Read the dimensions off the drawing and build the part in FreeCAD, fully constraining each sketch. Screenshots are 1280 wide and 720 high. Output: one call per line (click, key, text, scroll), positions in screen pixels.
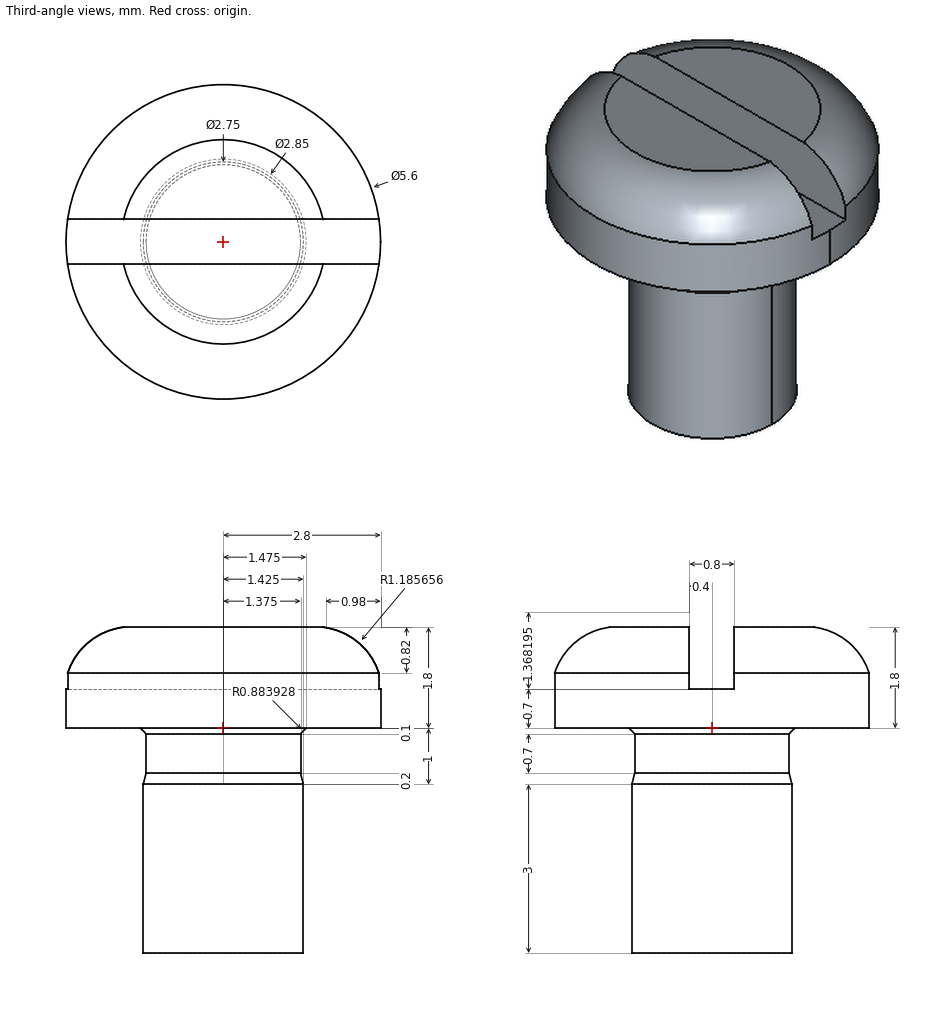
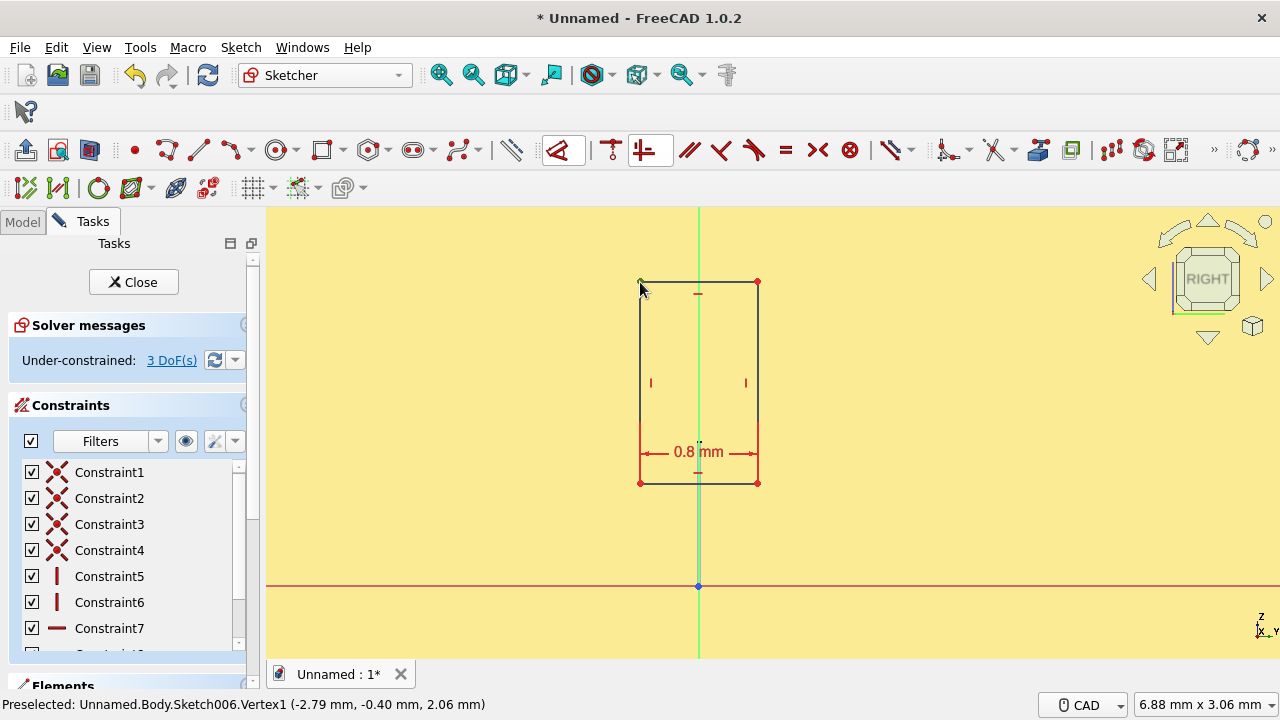
click(580, 150)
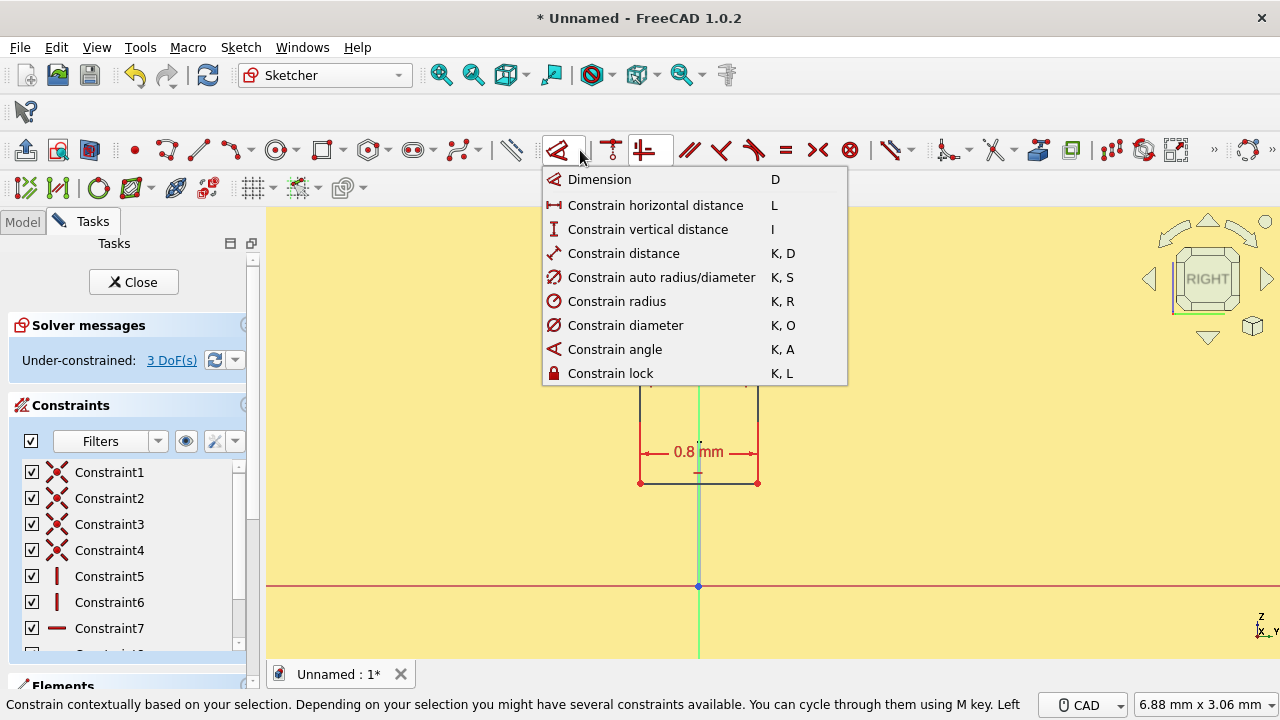
click(695, 205)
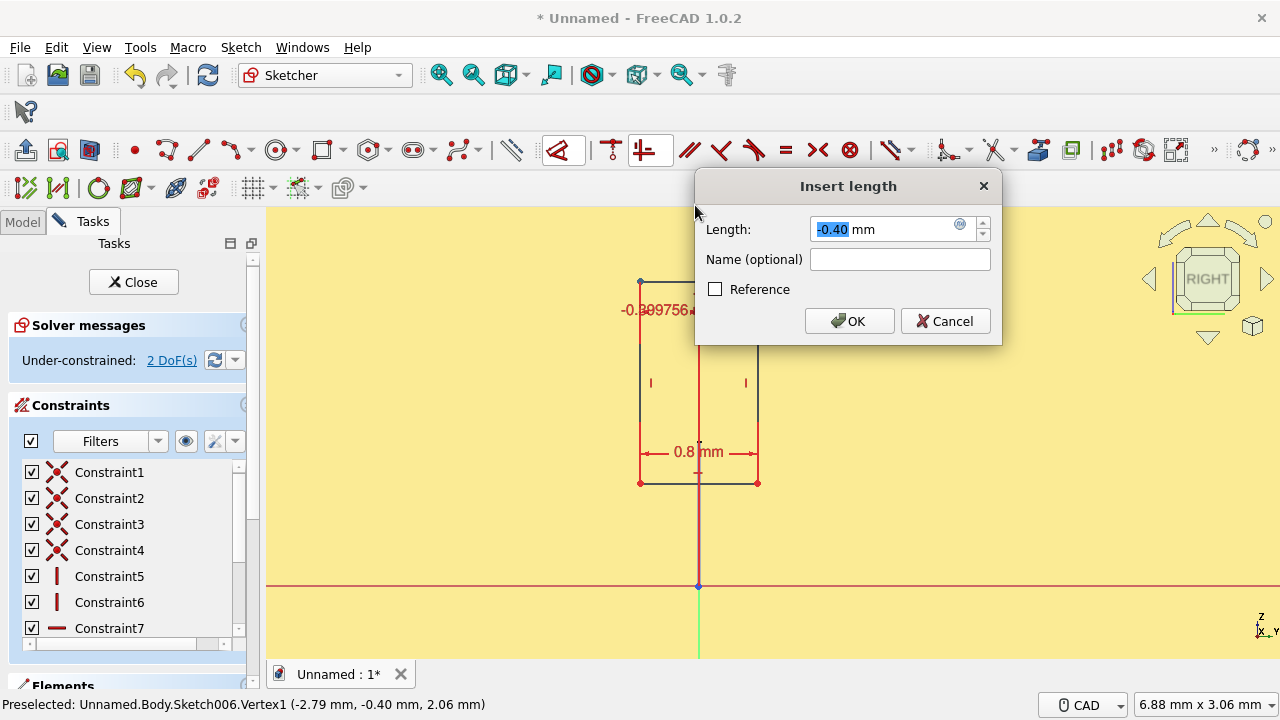
text(-0.4)
key(Return)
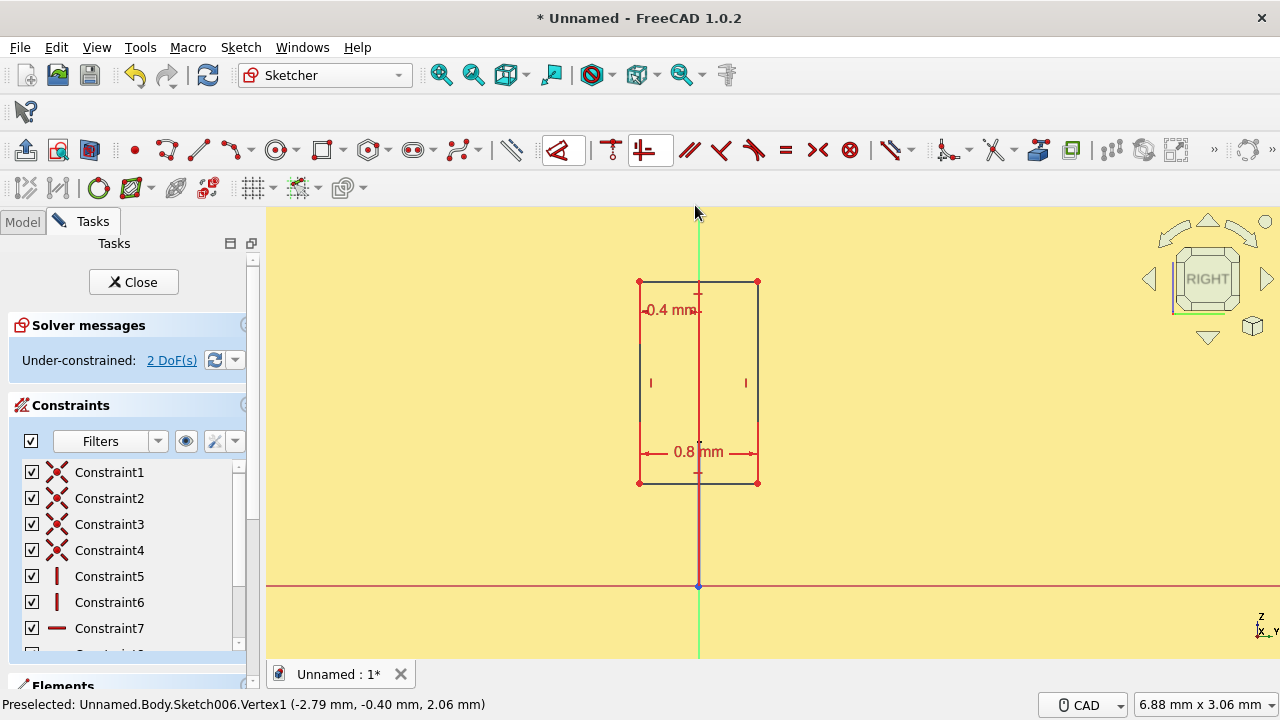
click(640, 484)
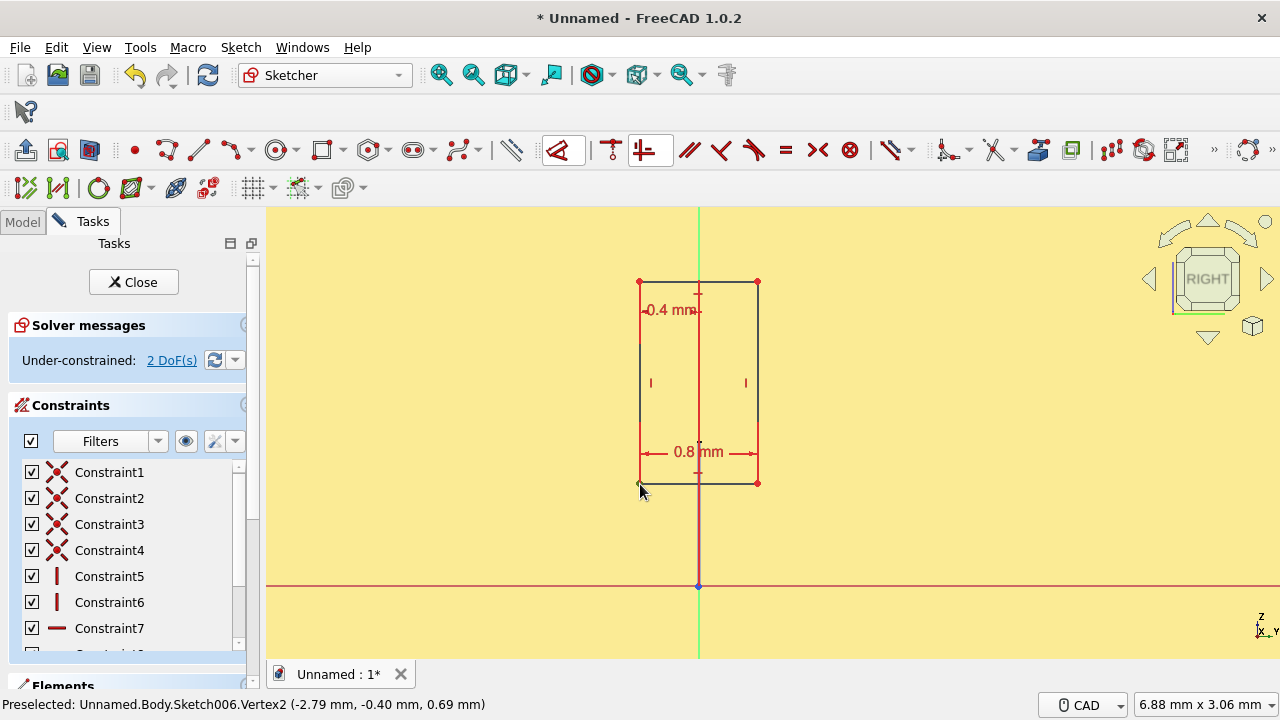
click(580, 150)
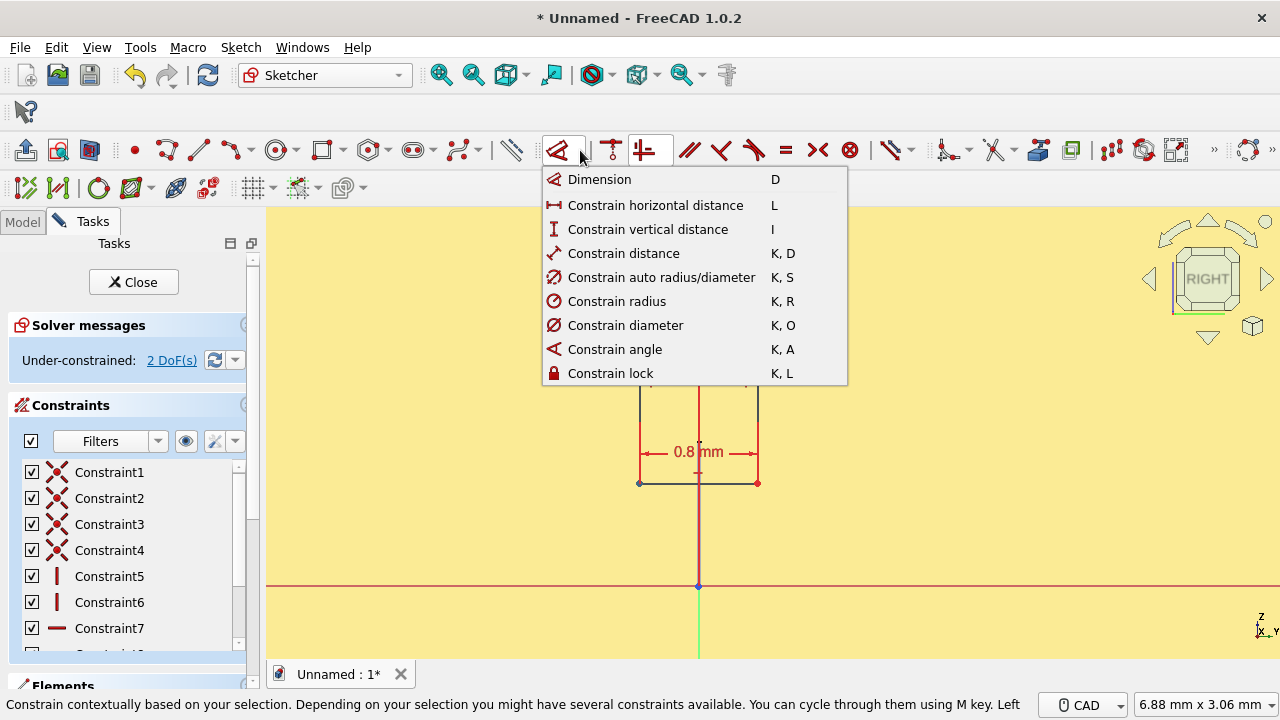
click(695, 229)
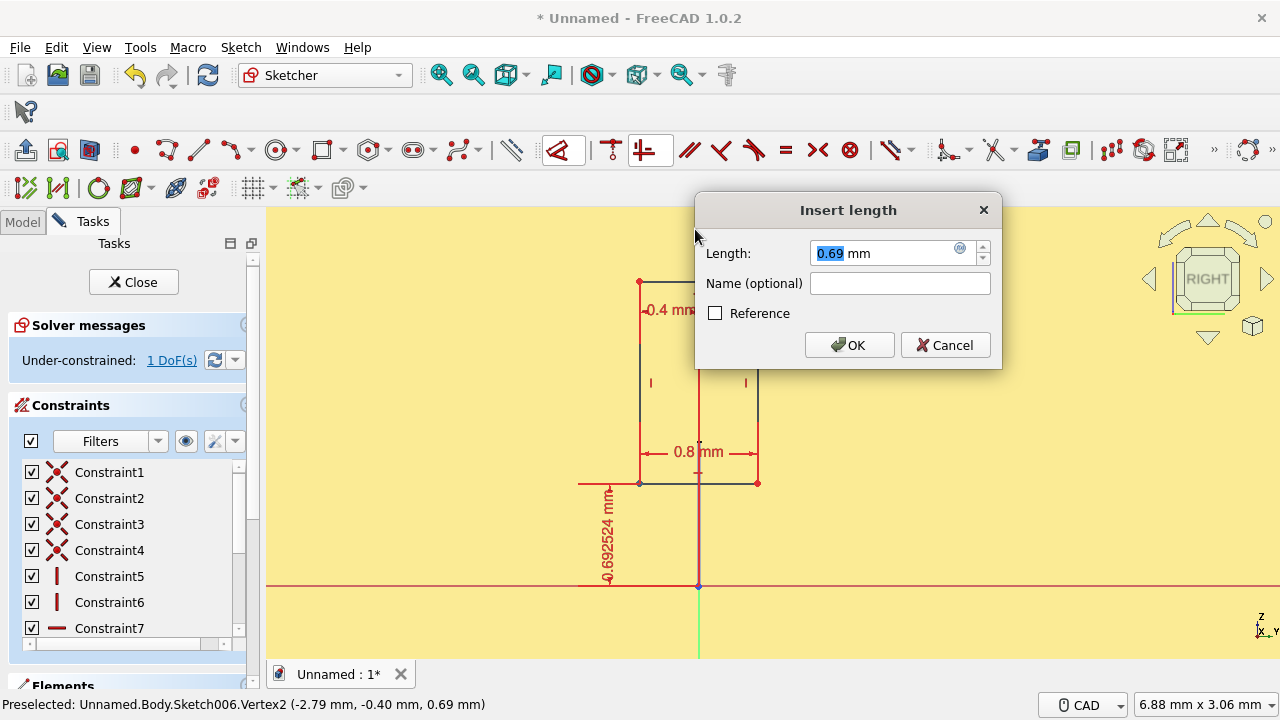
text(0.7)
key(Return)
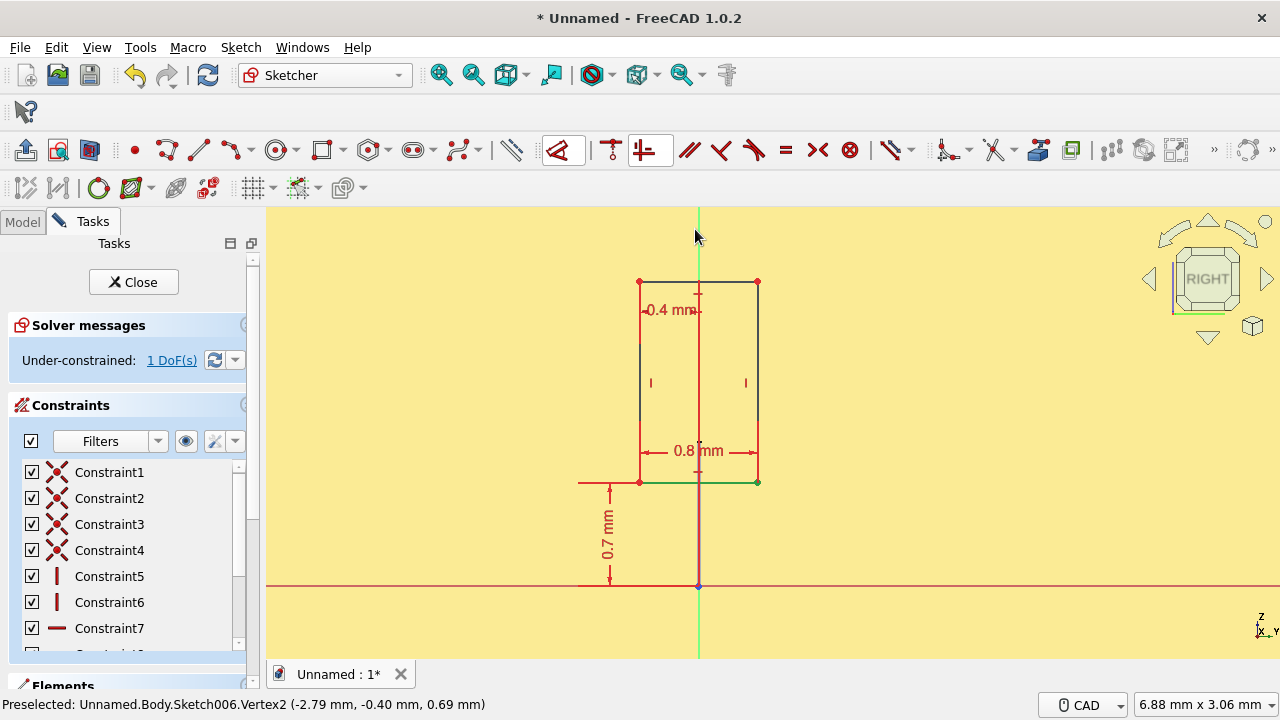
click(640, 342)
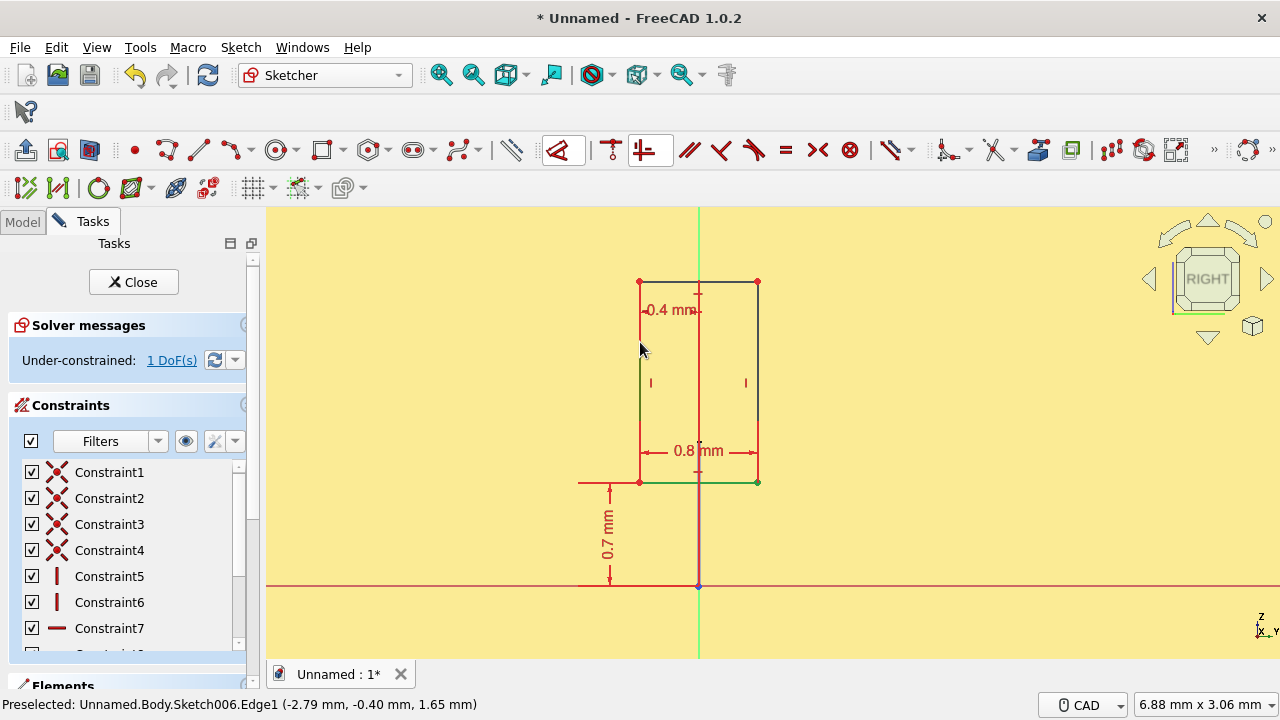
key(i)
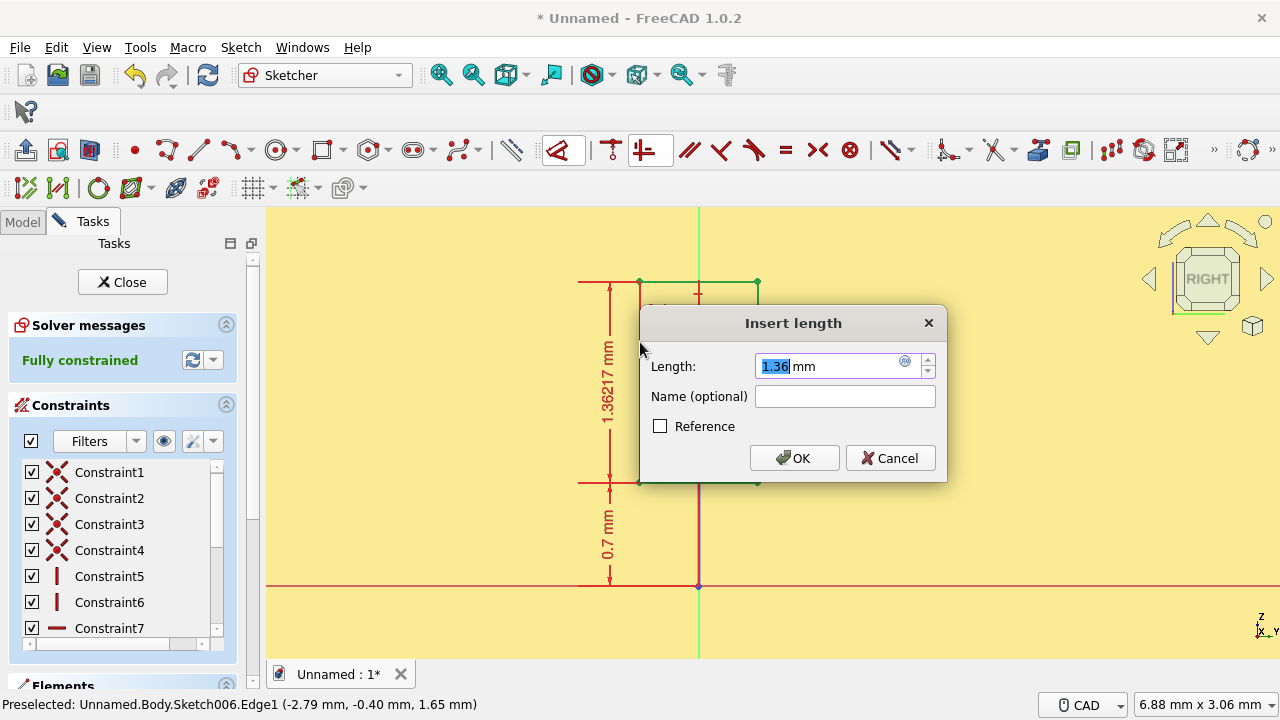
text(1.368195)
key(Return)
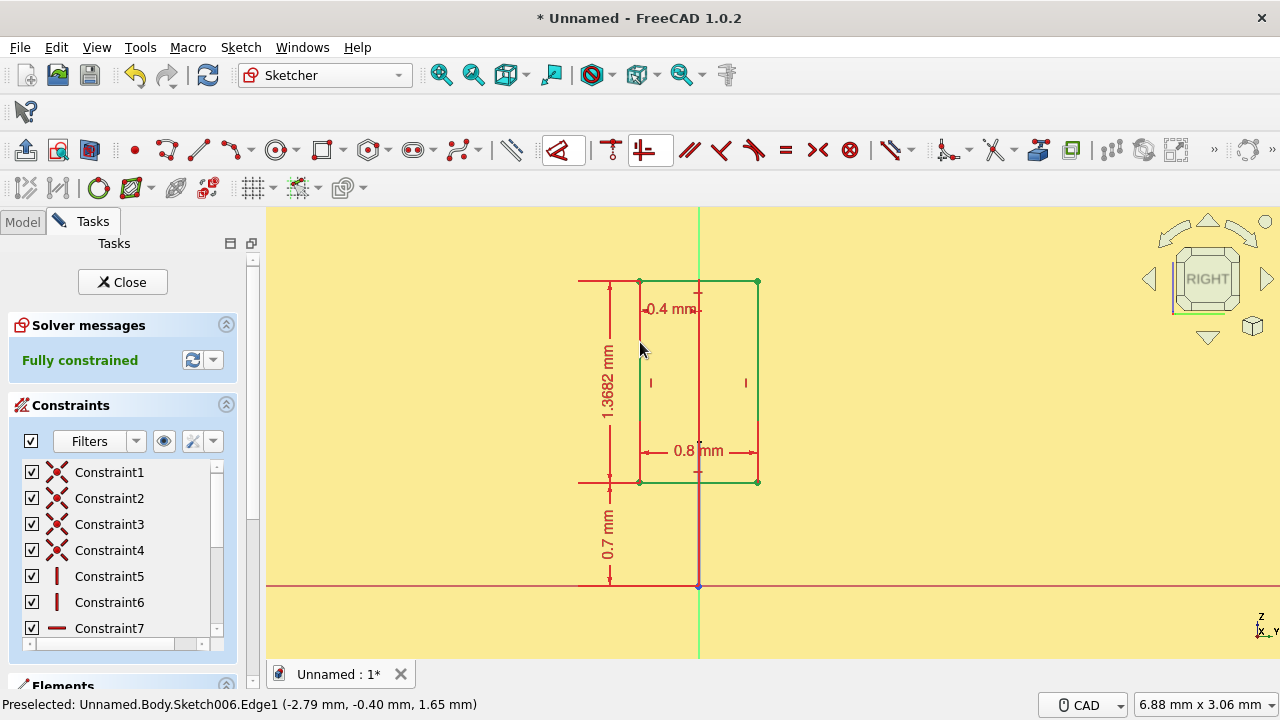
click(123, 282)